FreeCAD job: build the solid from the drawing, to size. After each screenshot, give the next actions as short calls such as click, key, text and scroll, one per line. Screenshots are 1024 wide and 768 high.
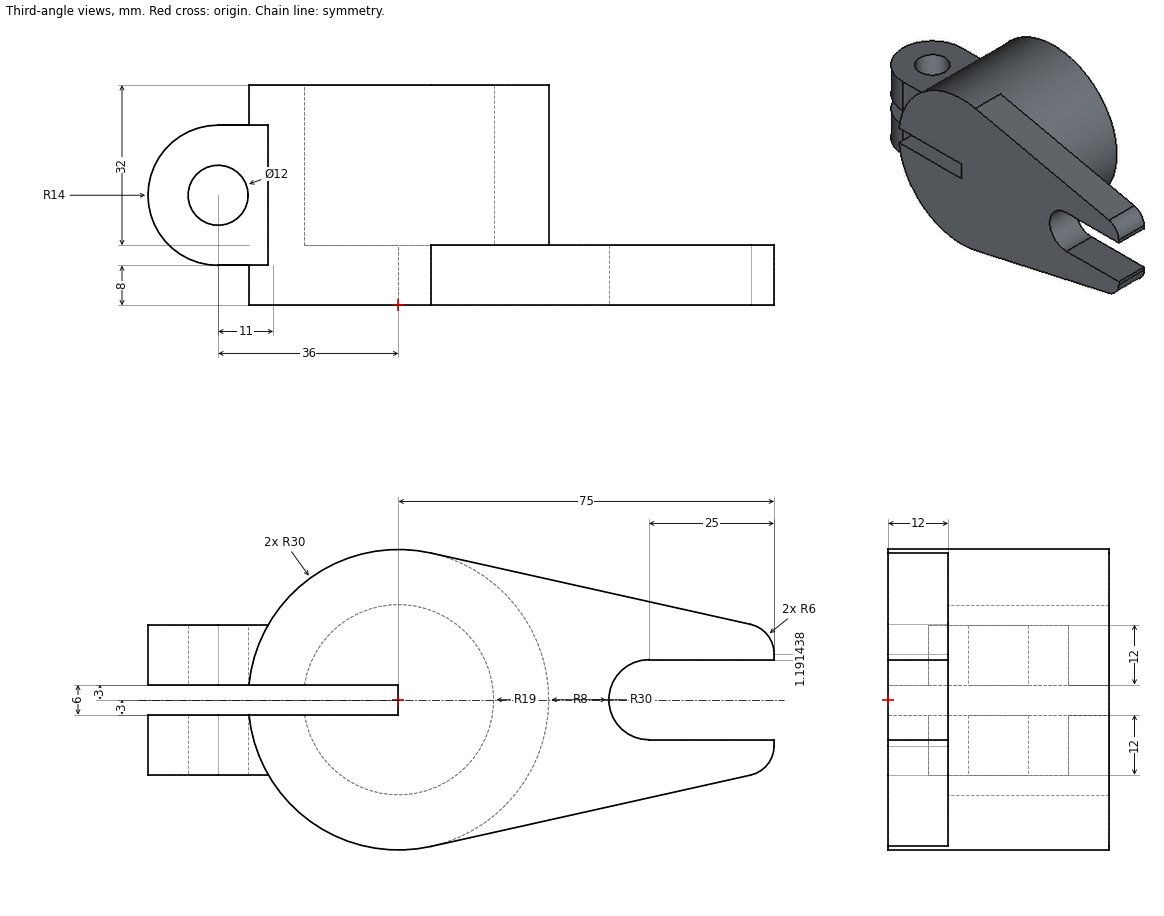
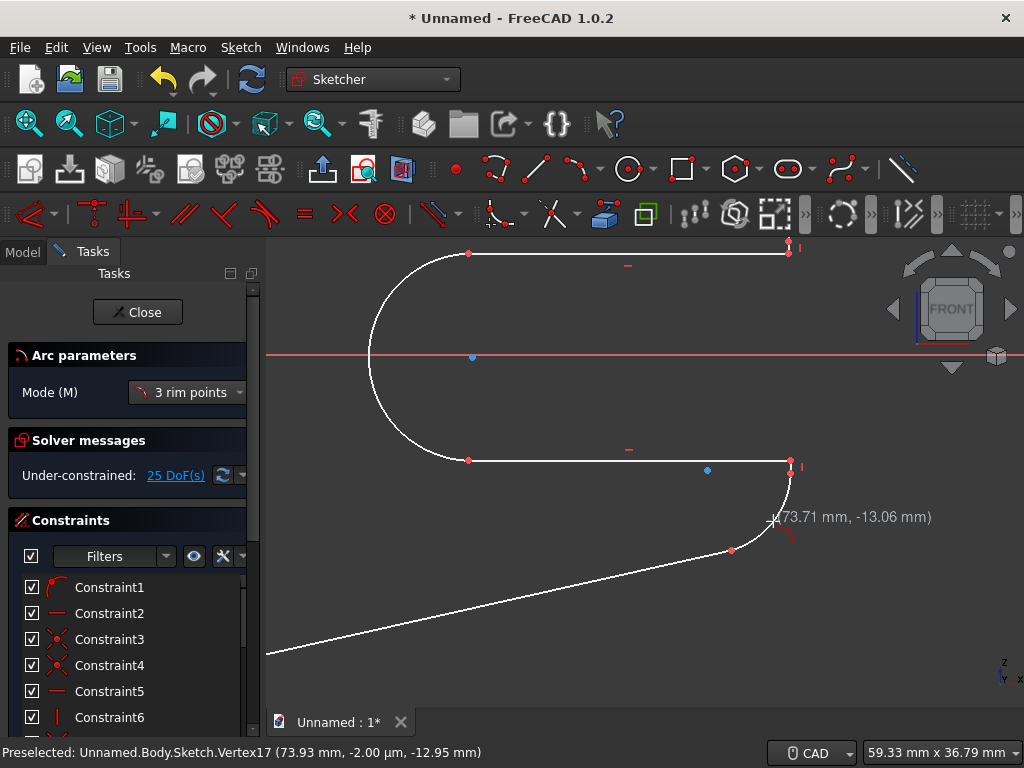
scroll(773, 522, down, 6)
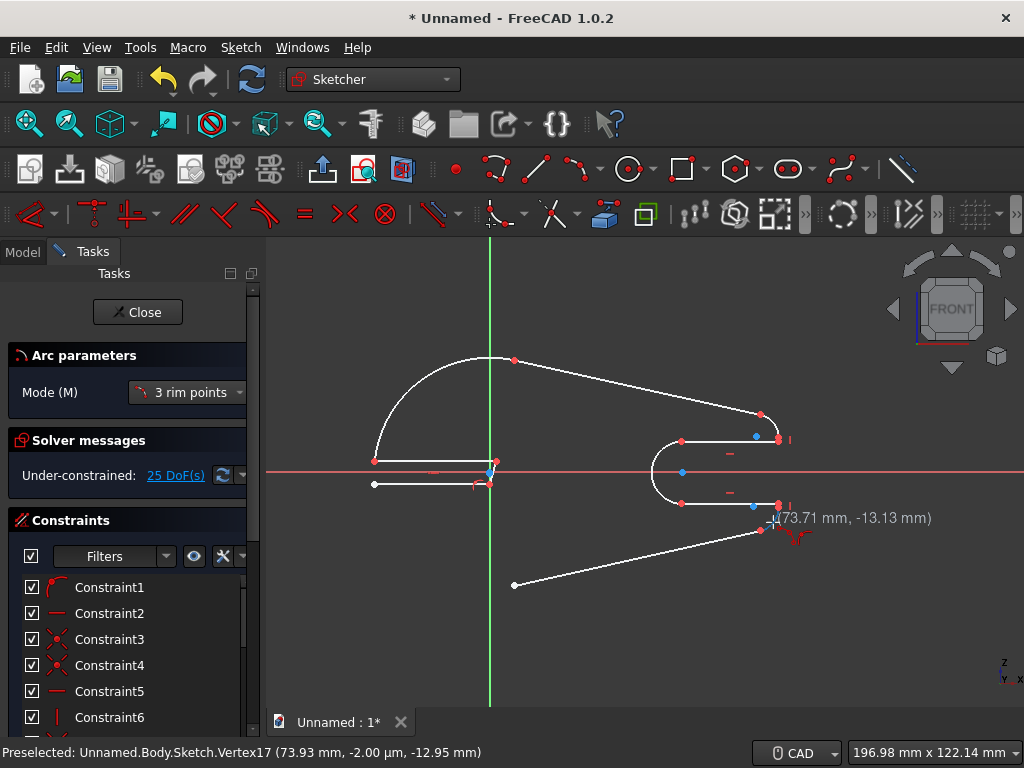
click(515, 586)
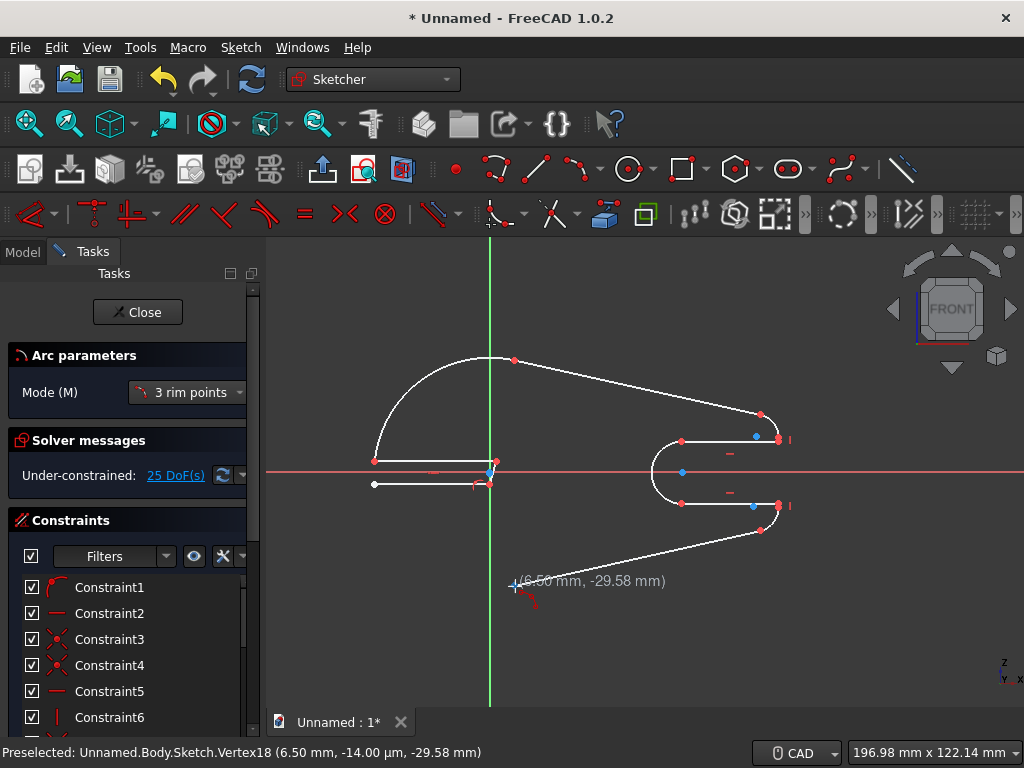
scroll(375, 484, up, 2)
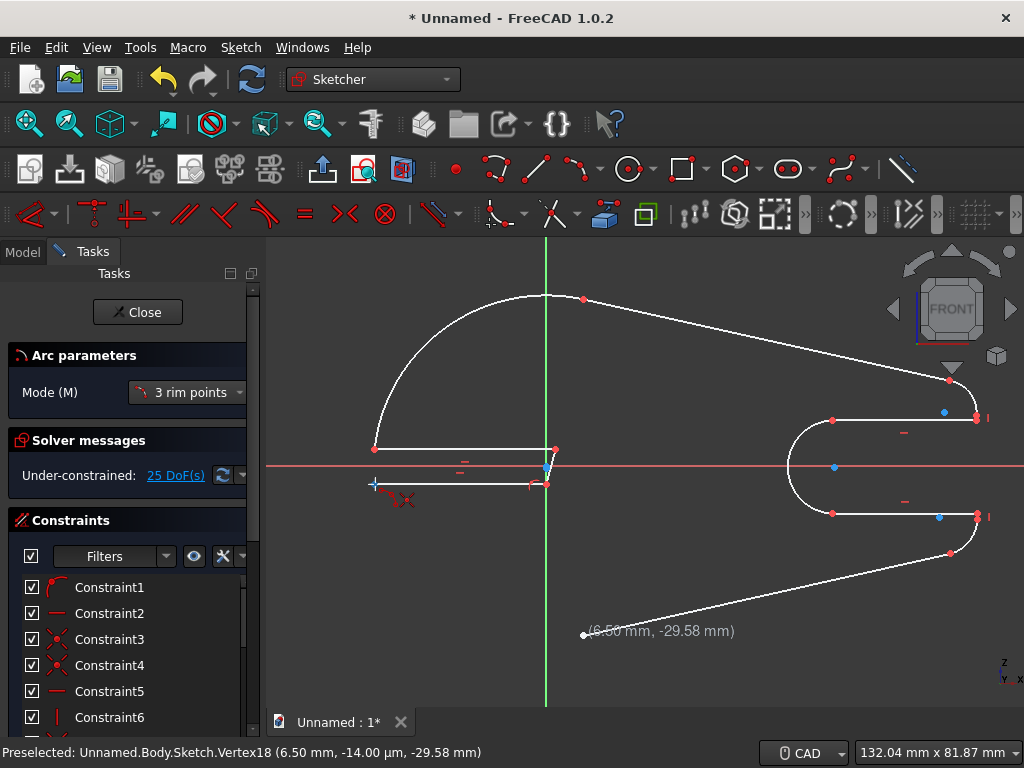
click(375, 484)
click(445, 606)
key(Escape)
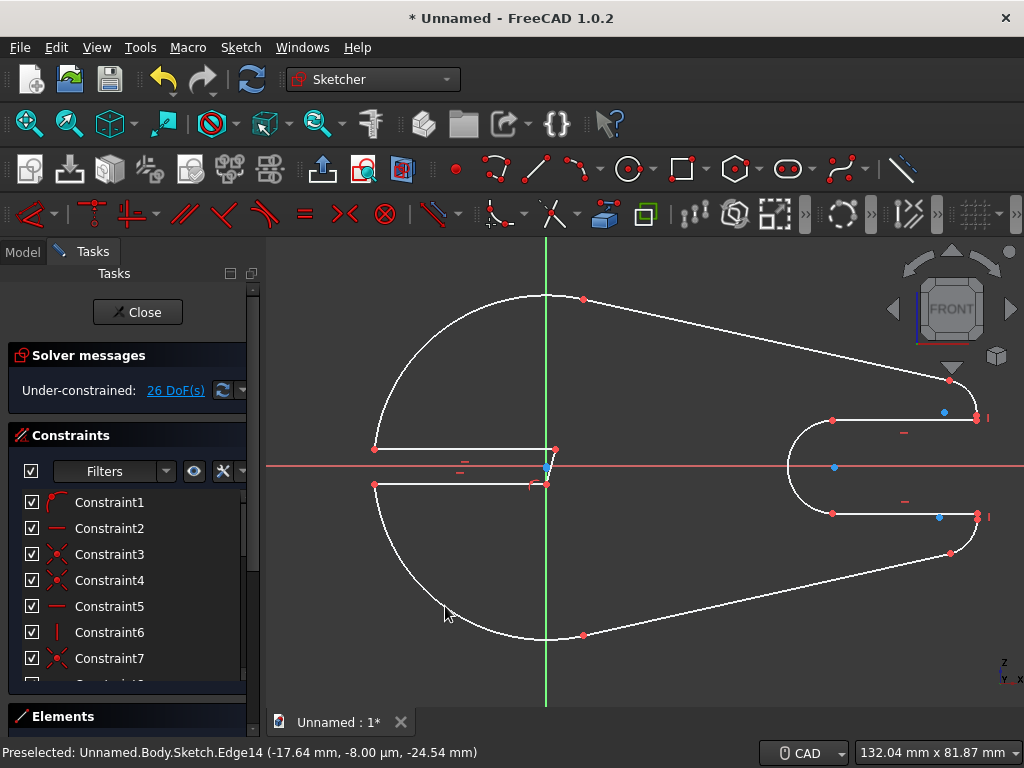
click(693, 324)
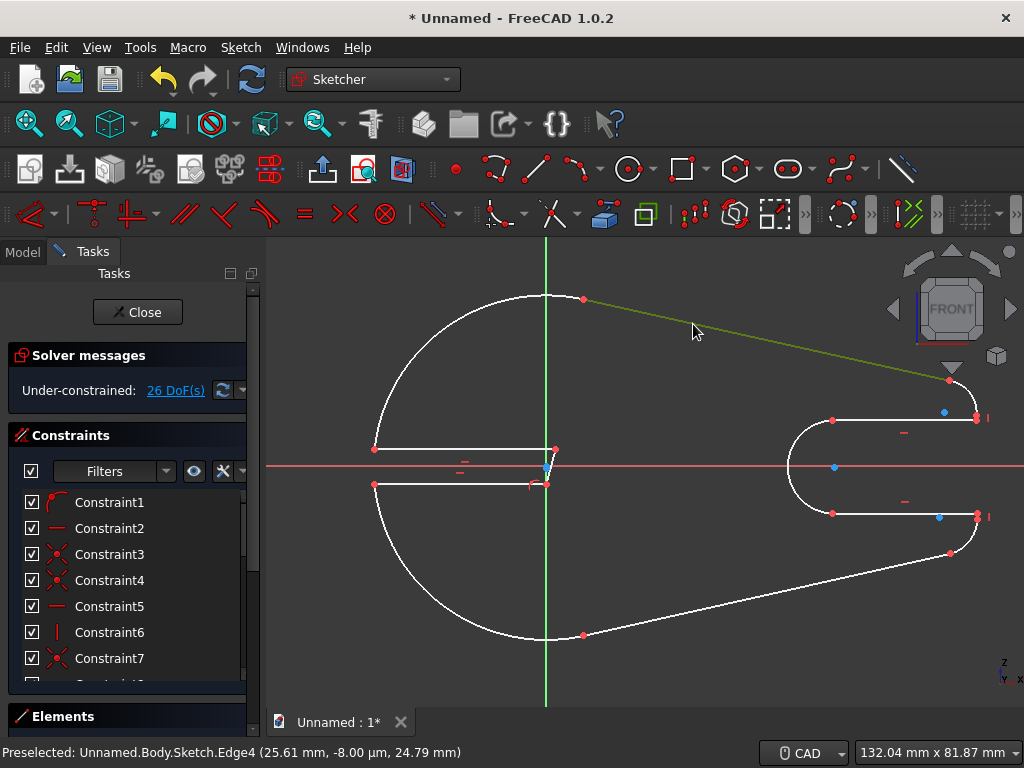
click(498, 302)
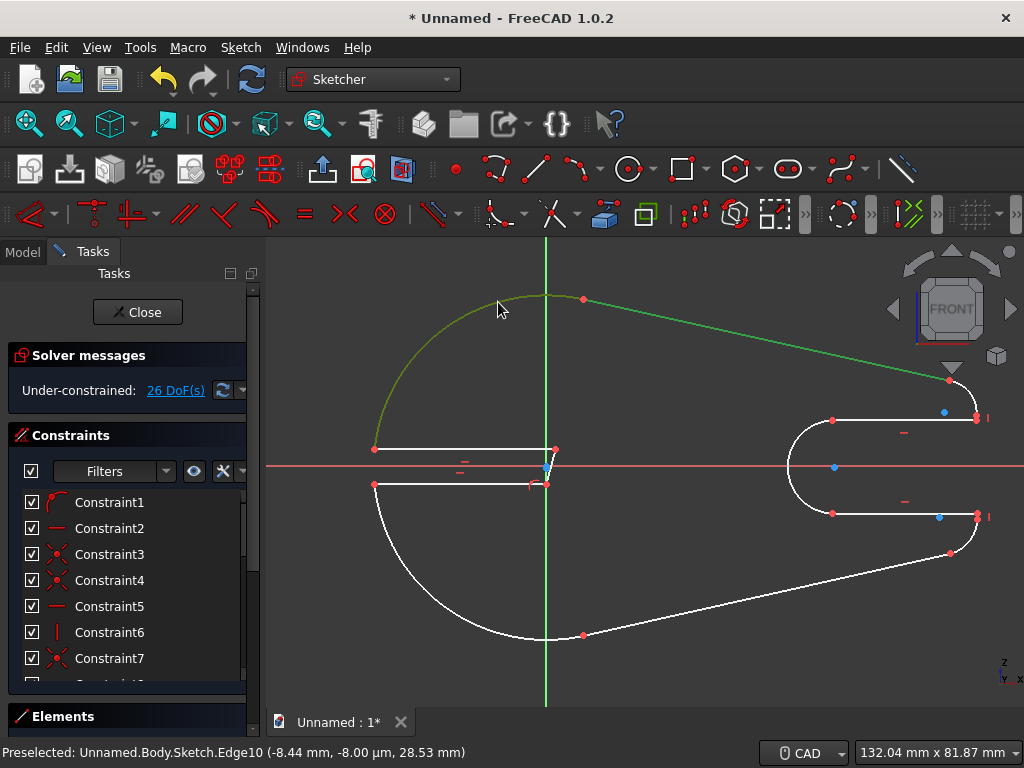
key(t)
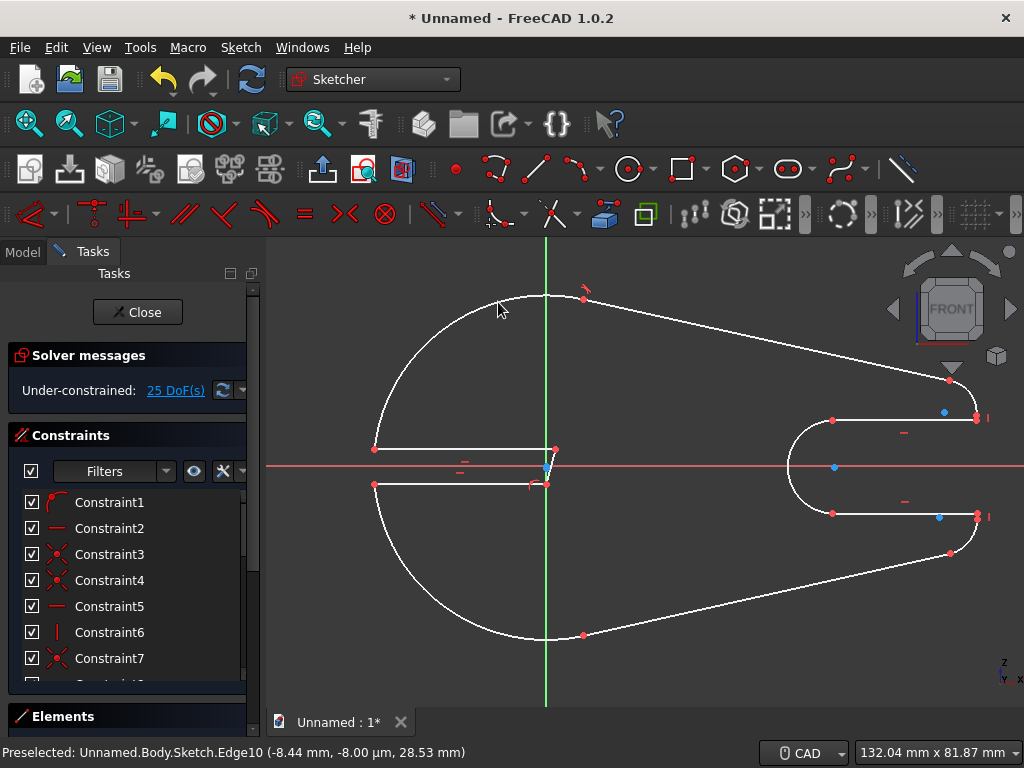
click(693, 324)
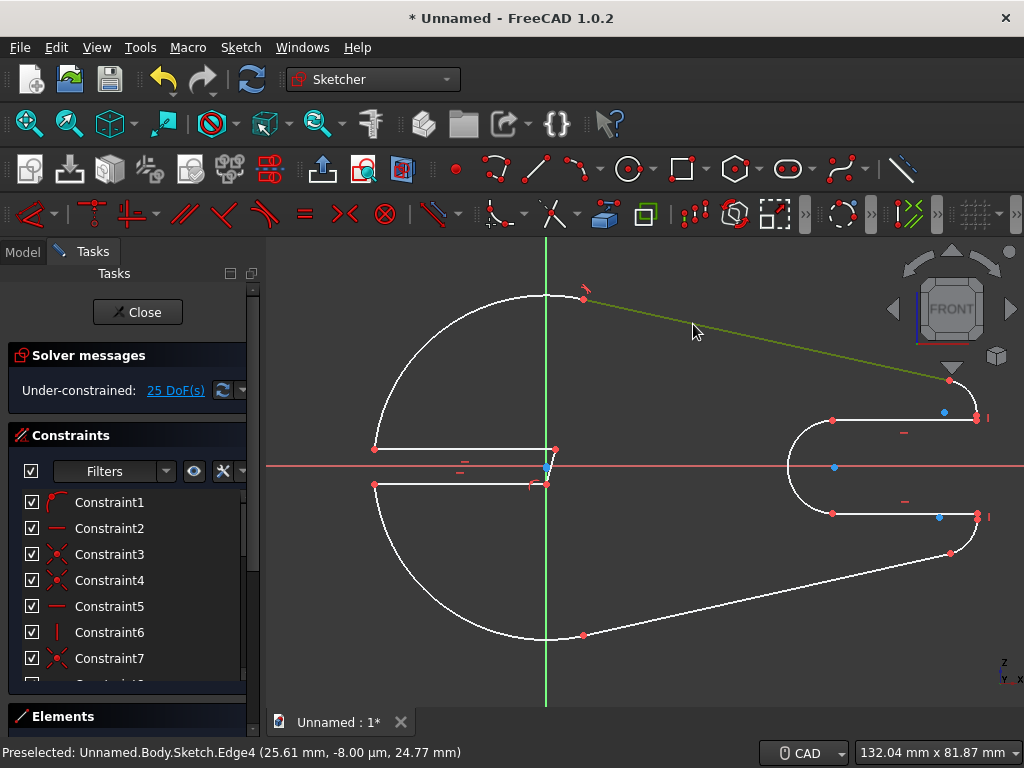
scroll(375, 484, down, 2)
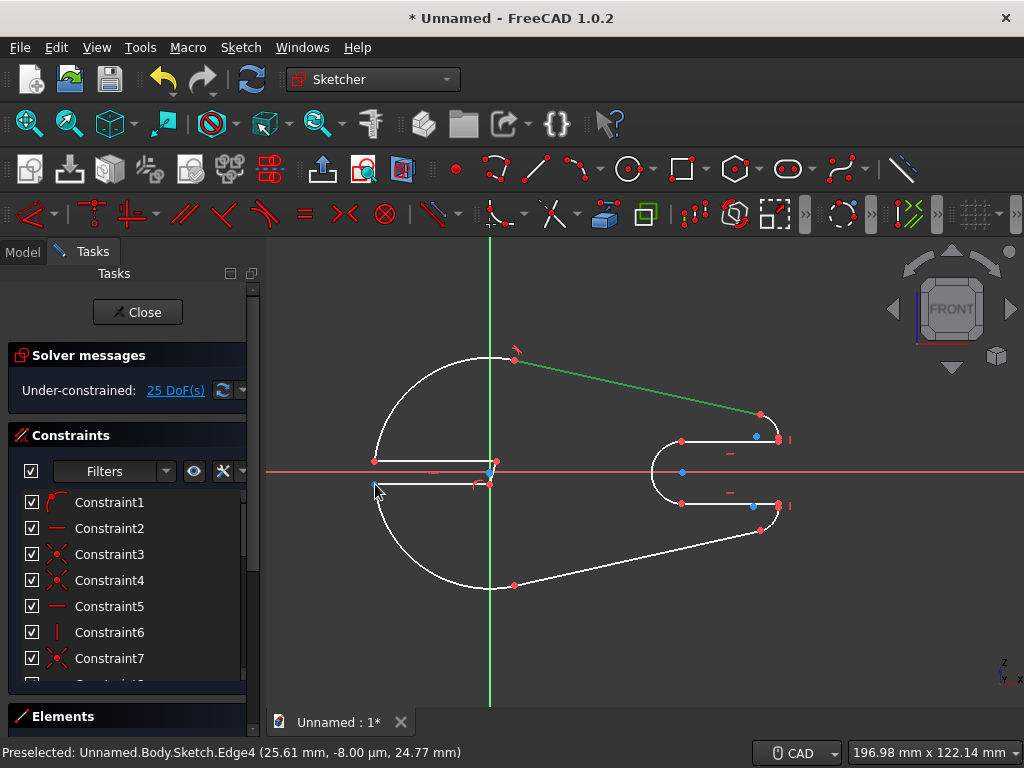
scroll(777, 429, up, 2)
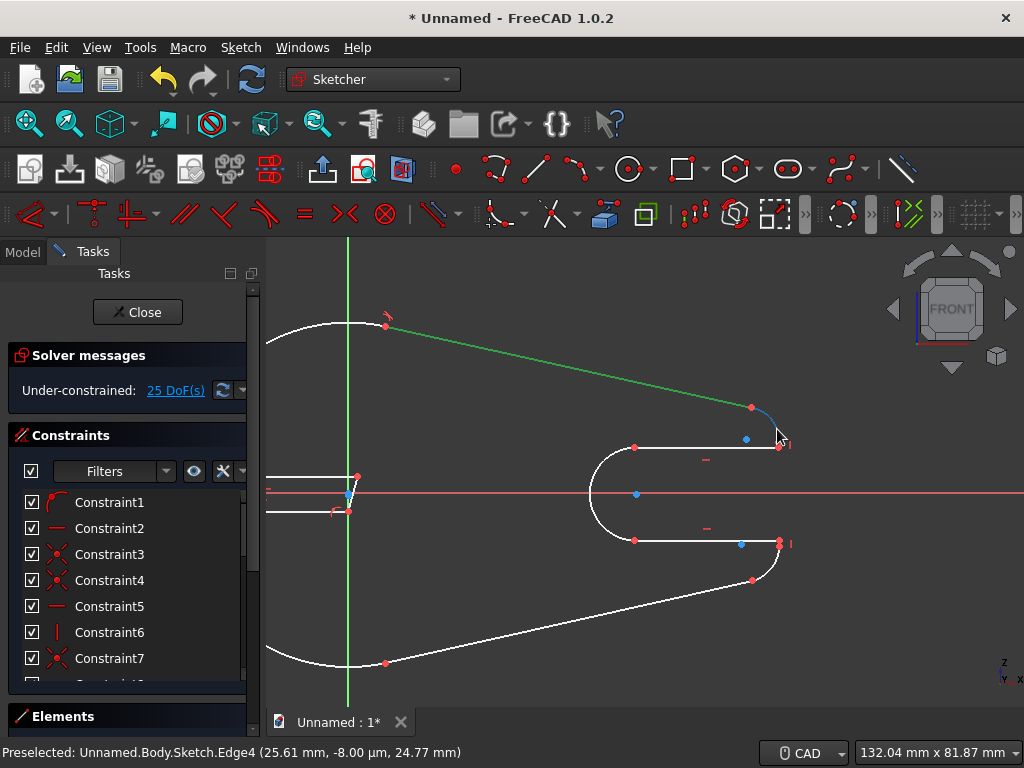
click(777, 428)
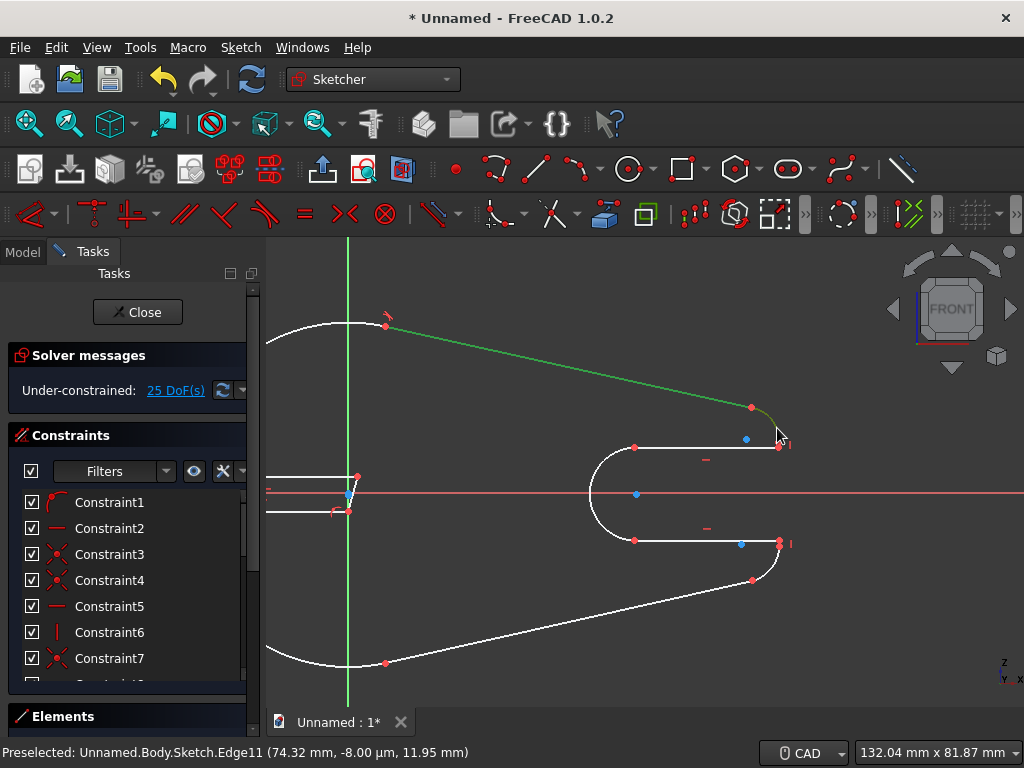
key(t)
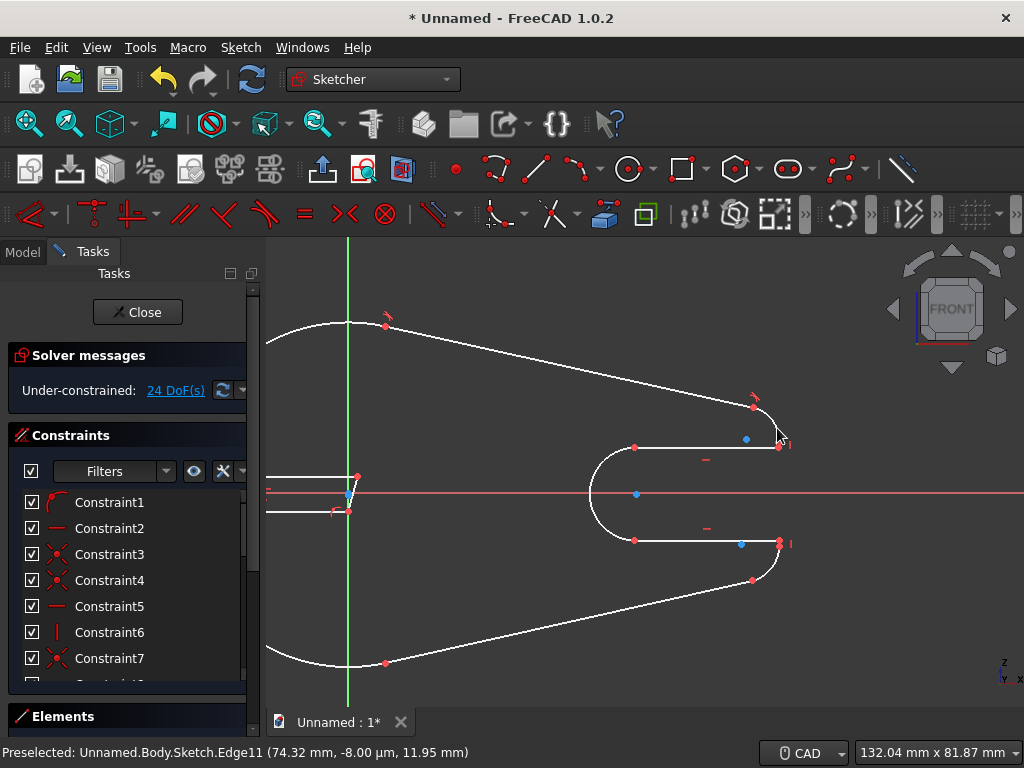
scroll(779, 445, up, 9)